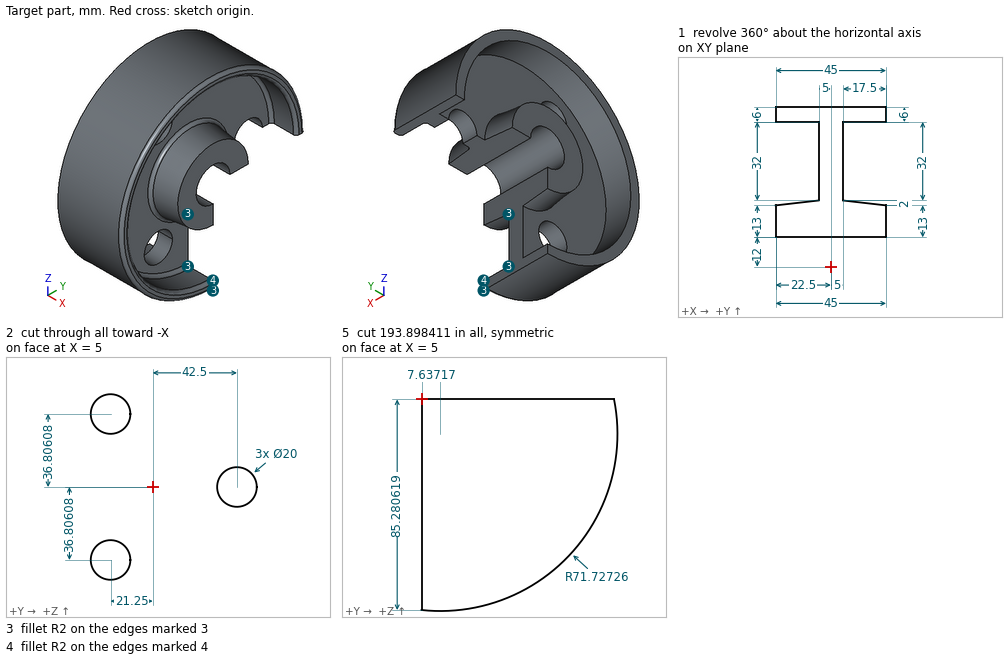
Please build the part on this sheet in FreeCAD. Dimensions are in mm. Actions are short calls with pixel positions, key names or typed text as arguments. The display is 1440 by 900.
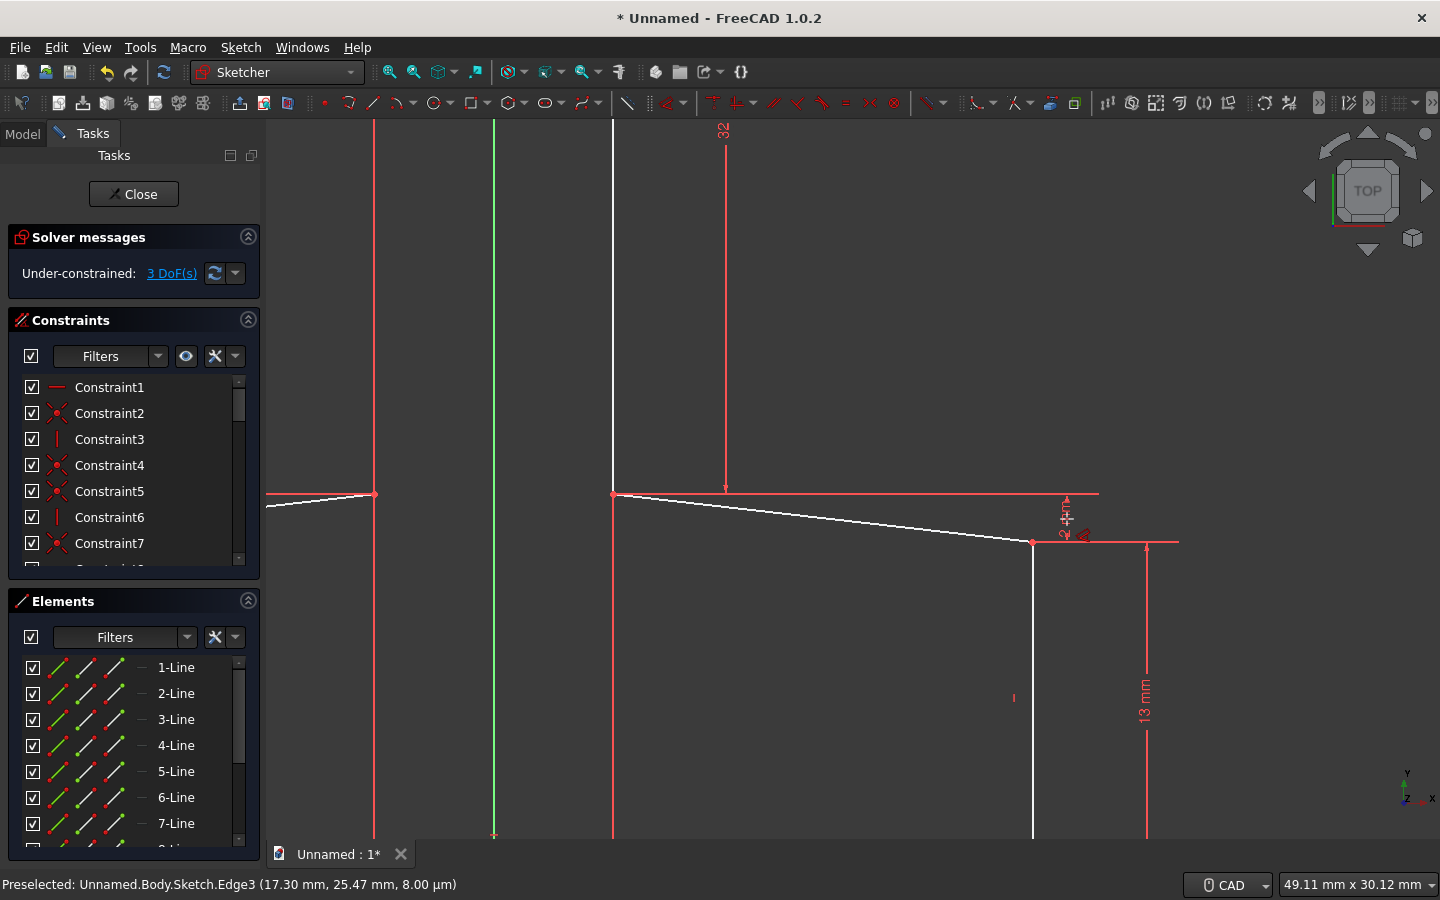
scroll(910, 530, down, 6)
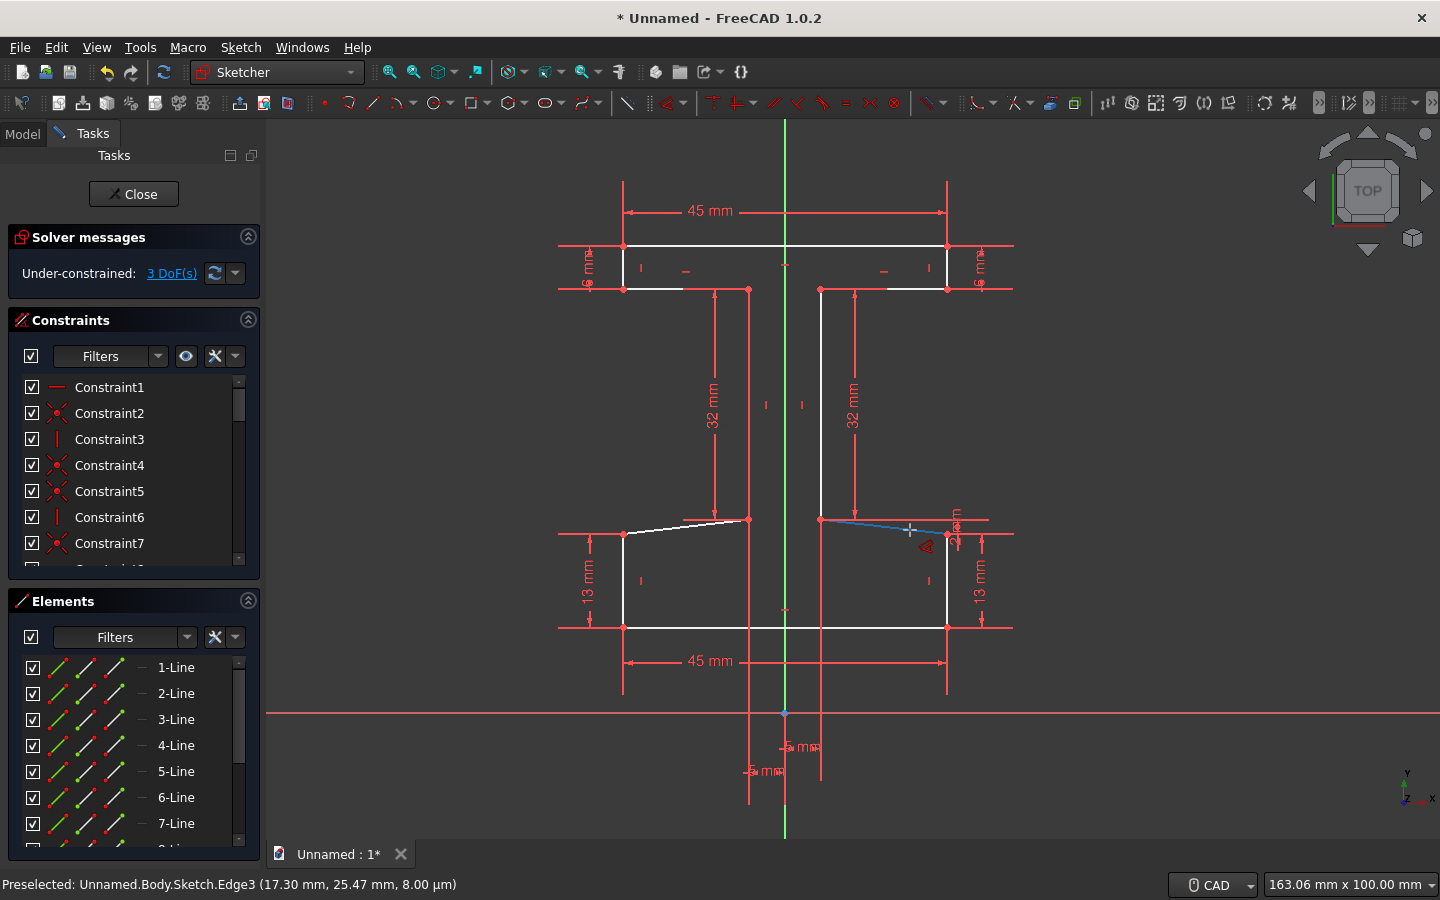
click(623, 628)
click(589, 671)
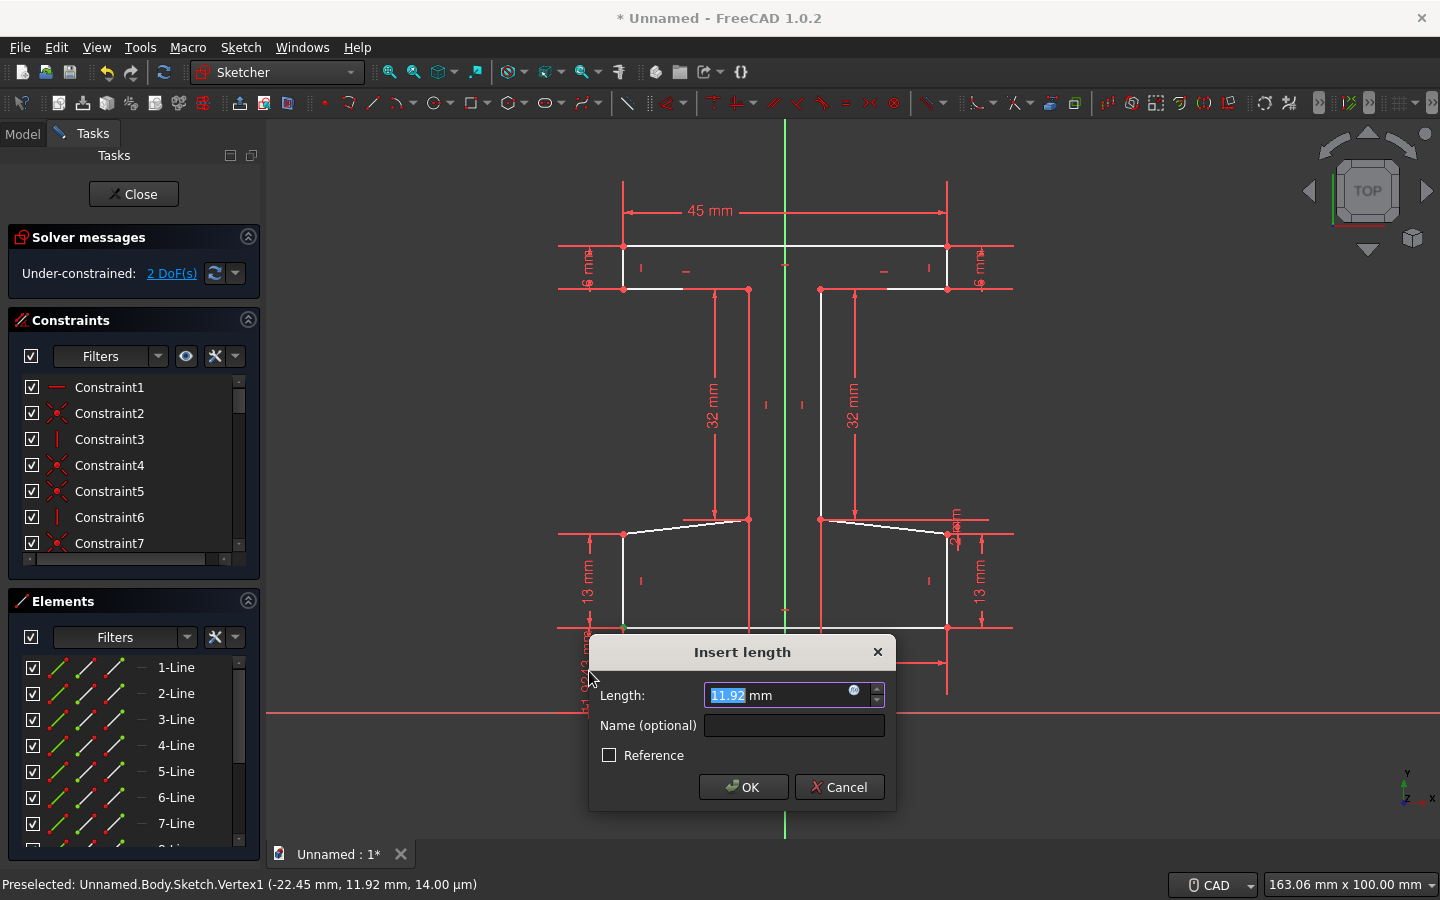
text(12)
key(Return)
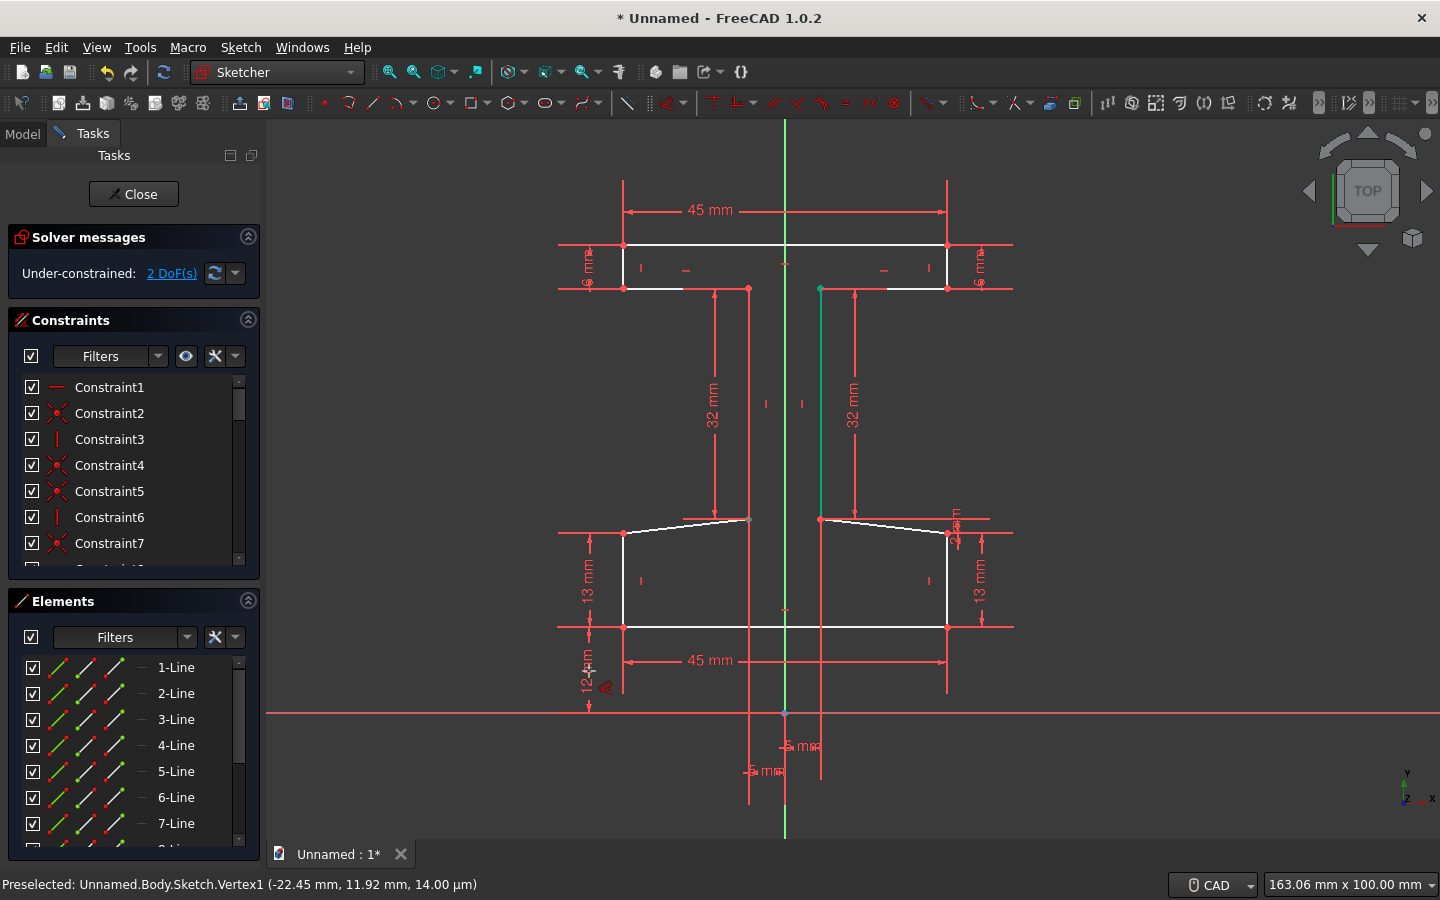
click(859, 289)
click(884, 323)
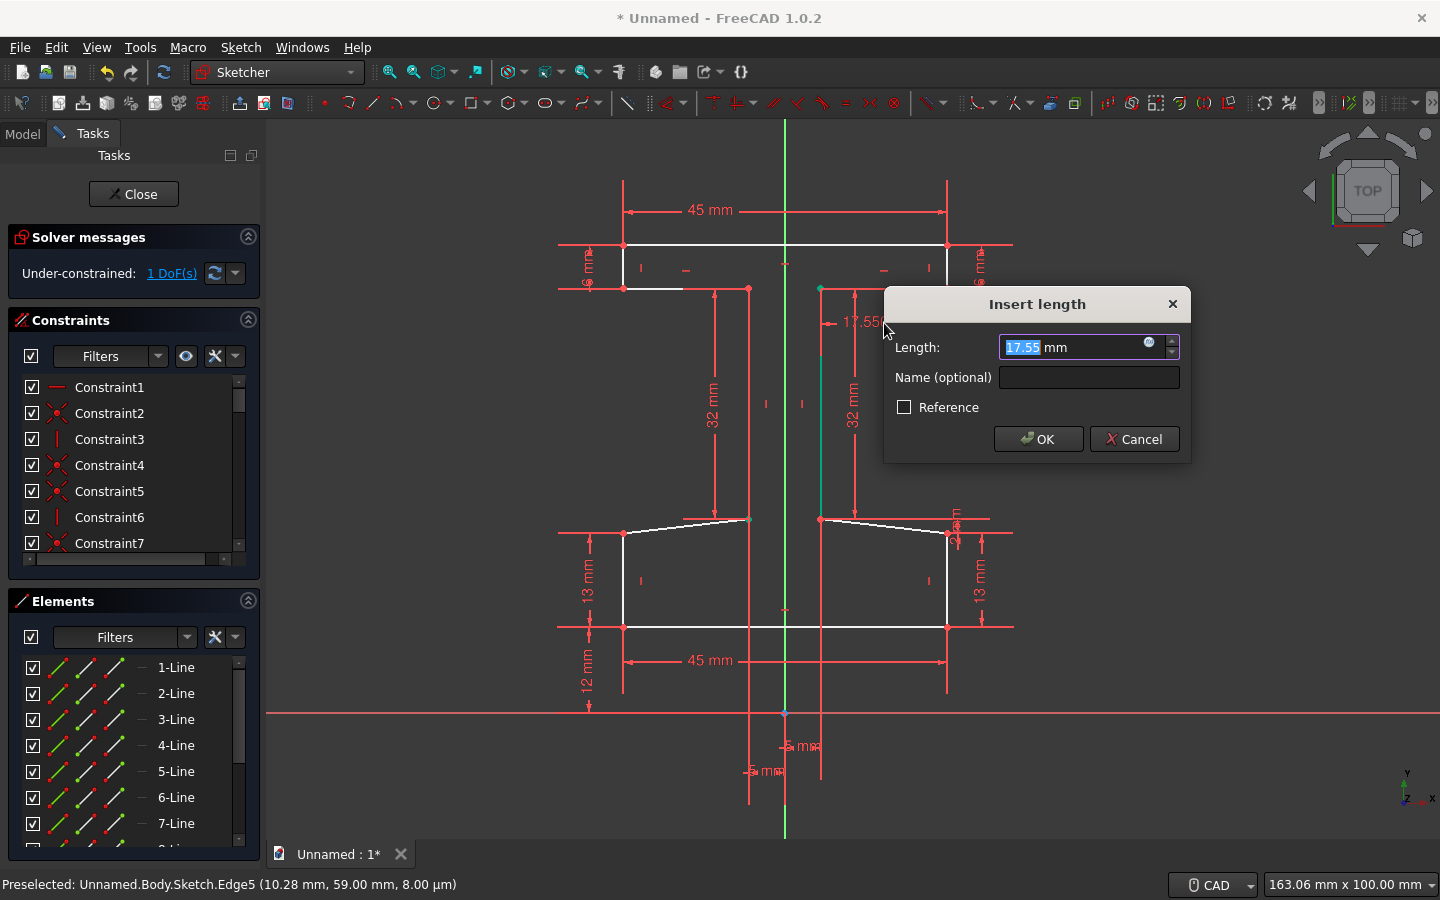
text(17.5)
key(Return)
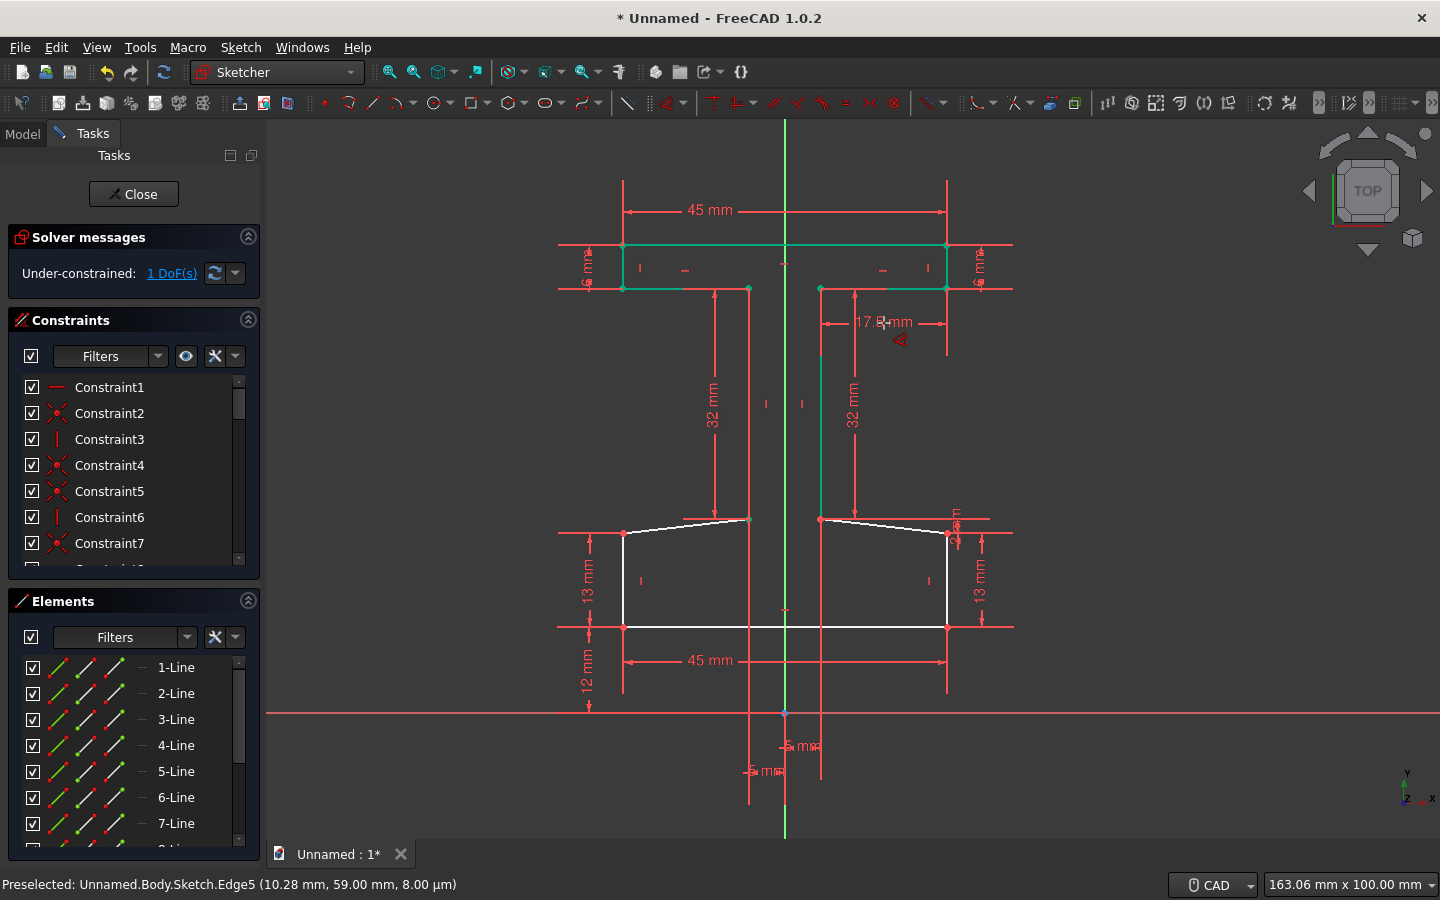
click(623, 627)
click(704, 747)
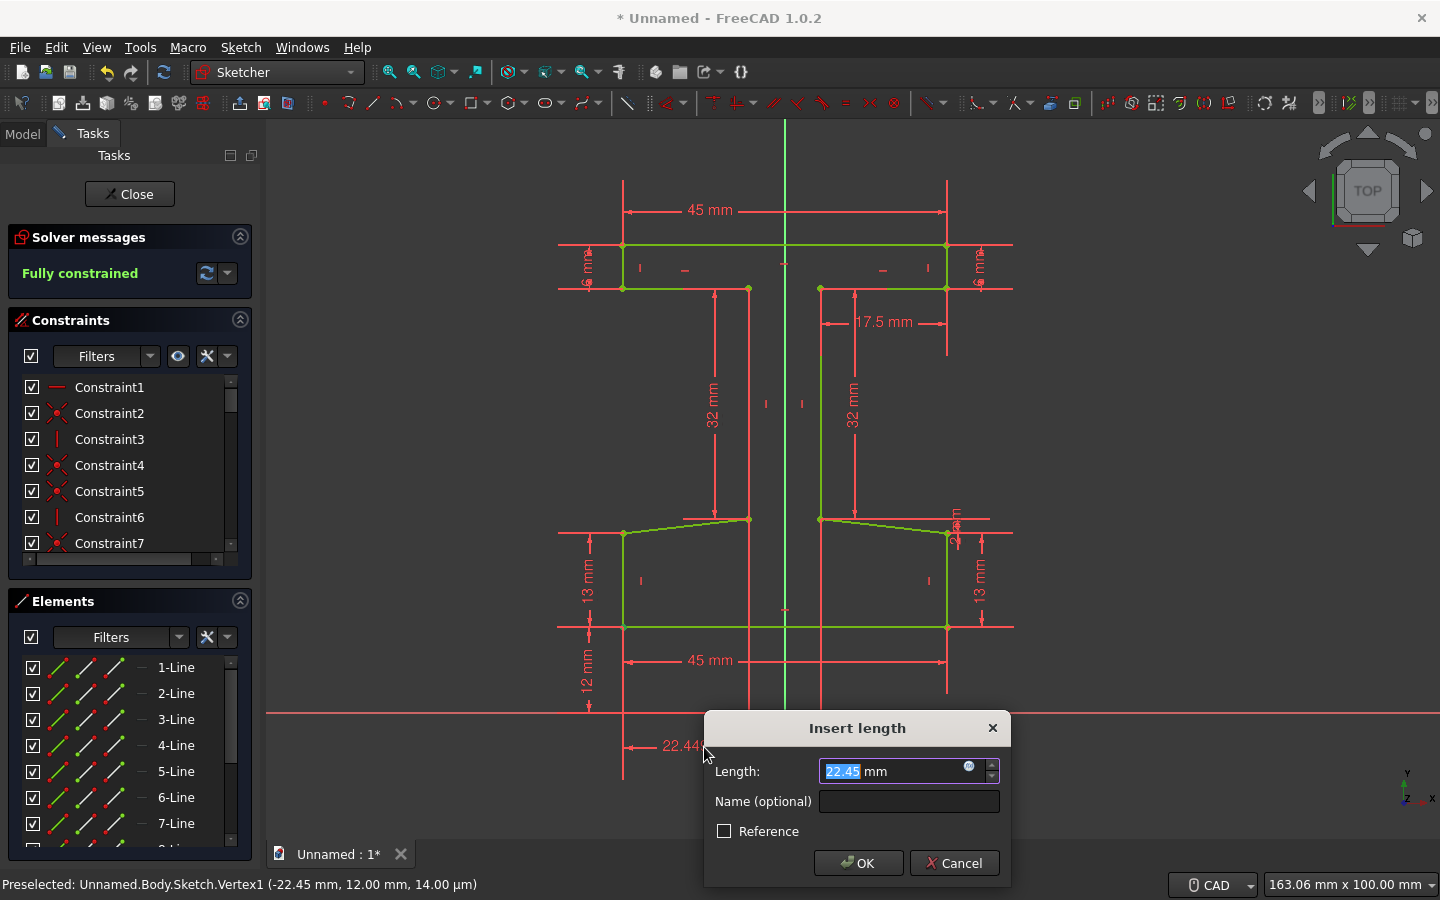
text(22.5)
key(Return)
key(Escape)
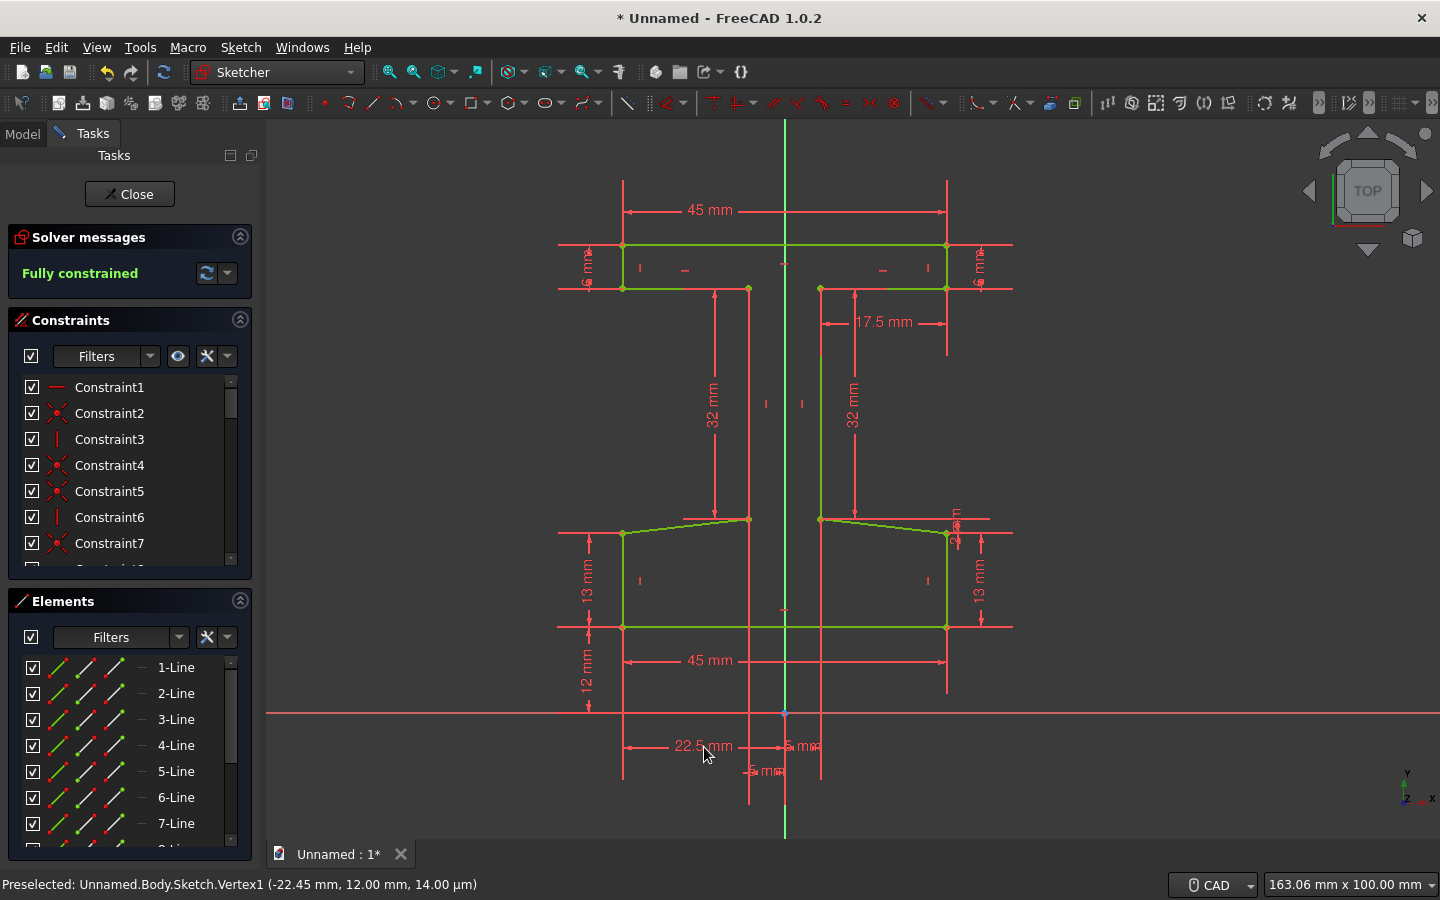
click(130, 194)